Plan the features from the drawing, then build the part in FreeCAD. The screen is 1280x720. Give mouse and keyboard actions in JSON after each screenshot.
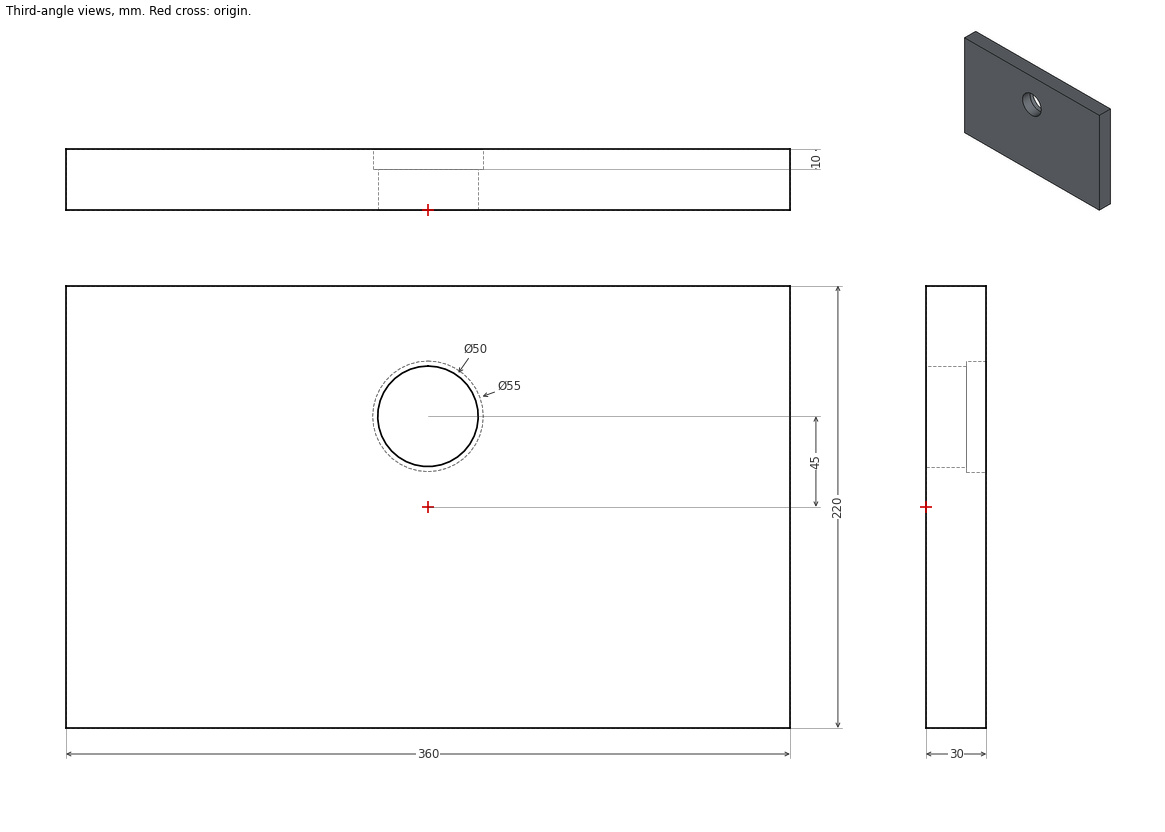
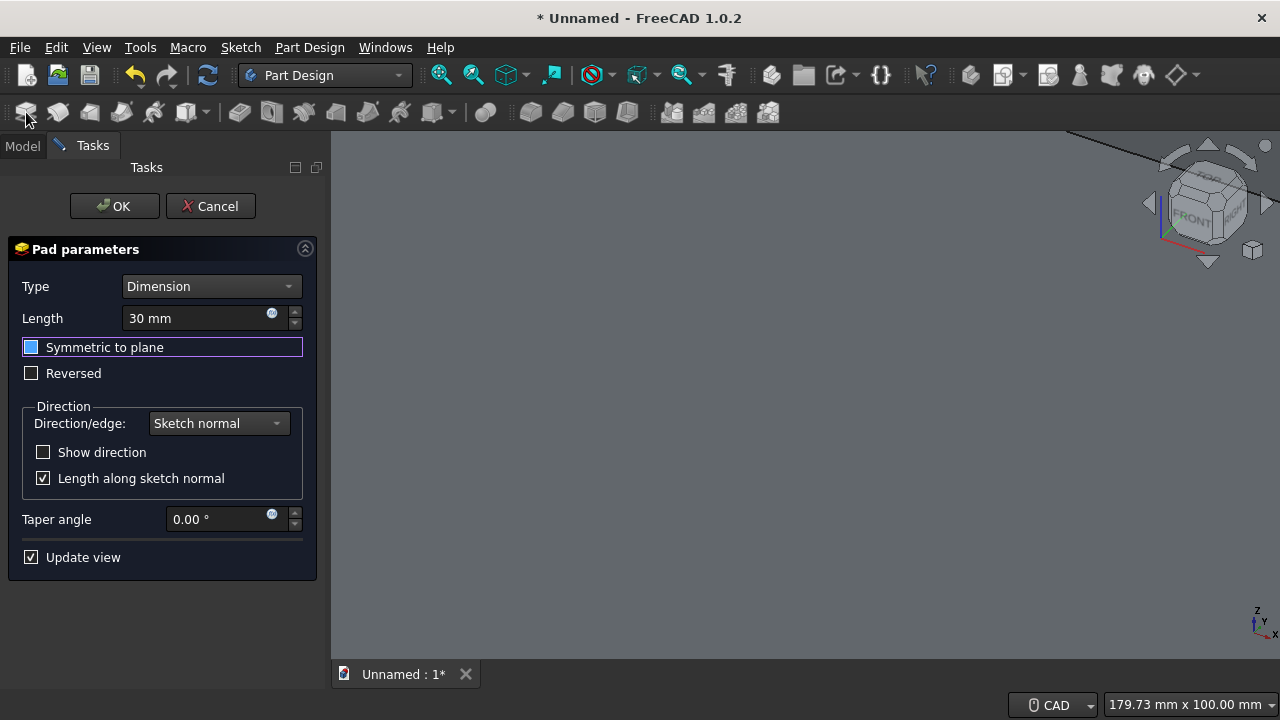
{"action": "left_click", "coordinate": [30, 373]}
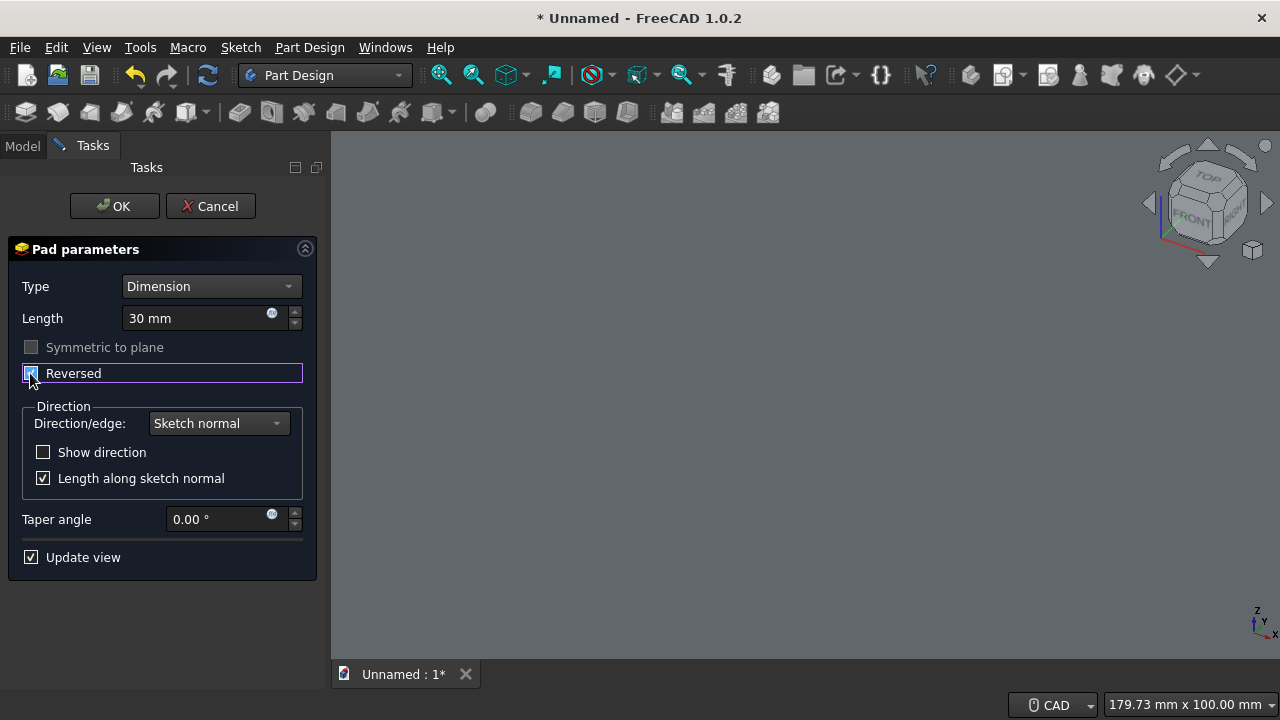
{"action": "left_click", "coordinate": [115, 206]}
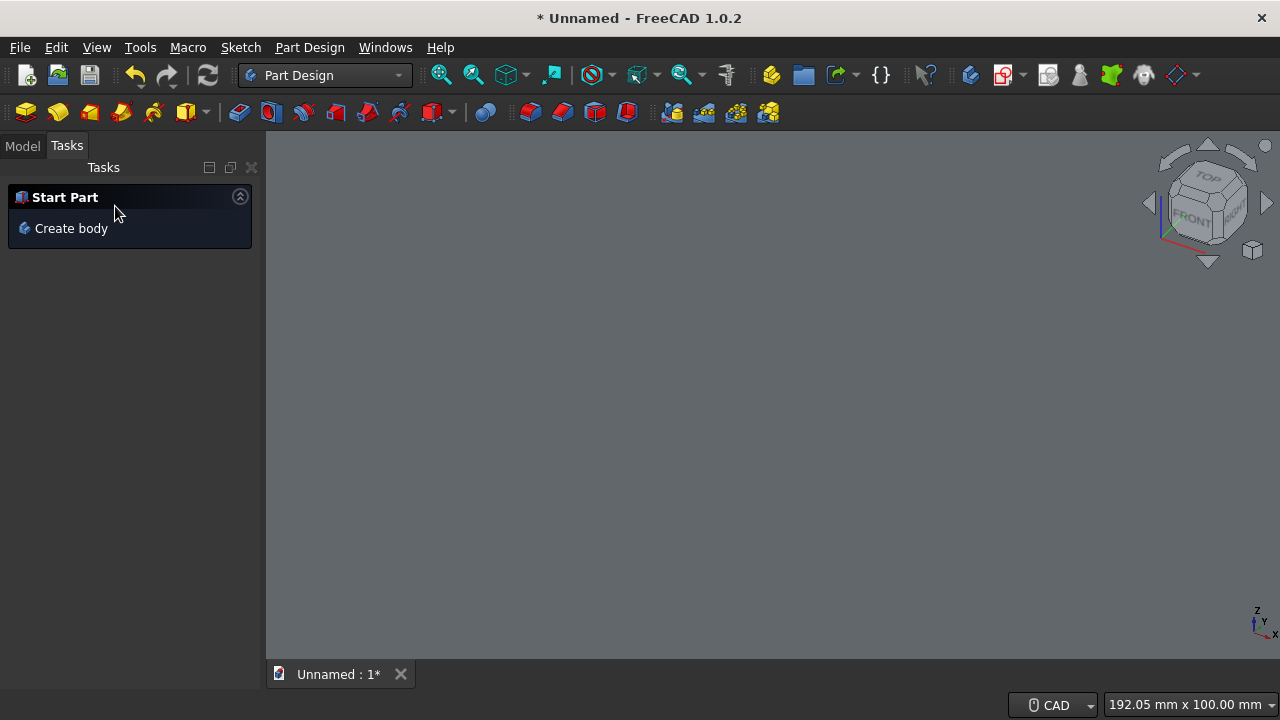
{"action": "key", "text": "v f"}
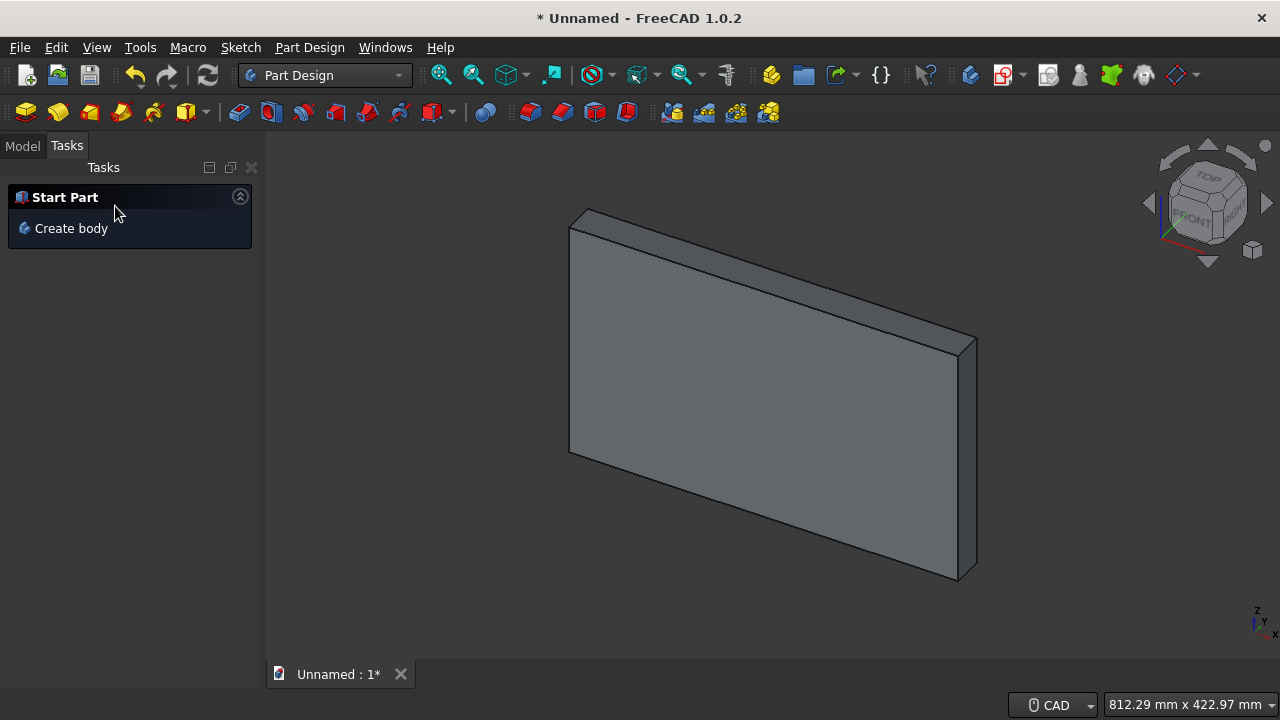
{"action": "key", "text": "4"}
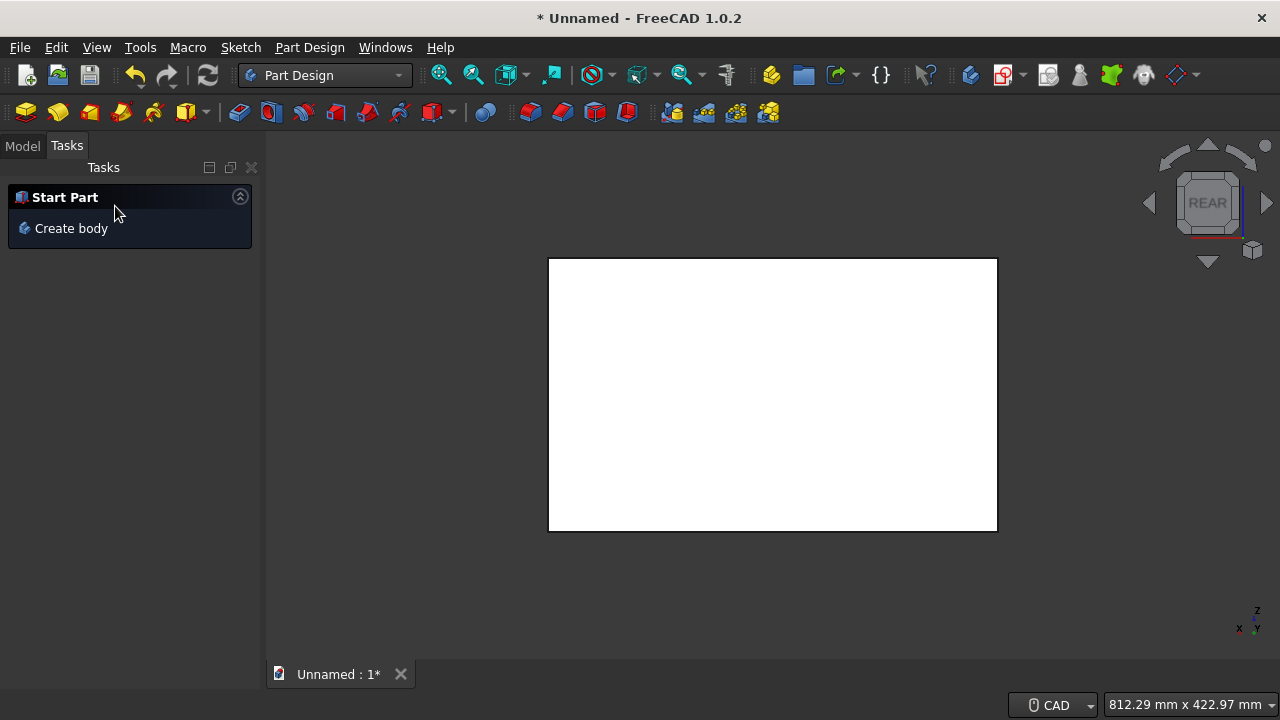
{"action": "left_click", "coordinate": [709, 394]}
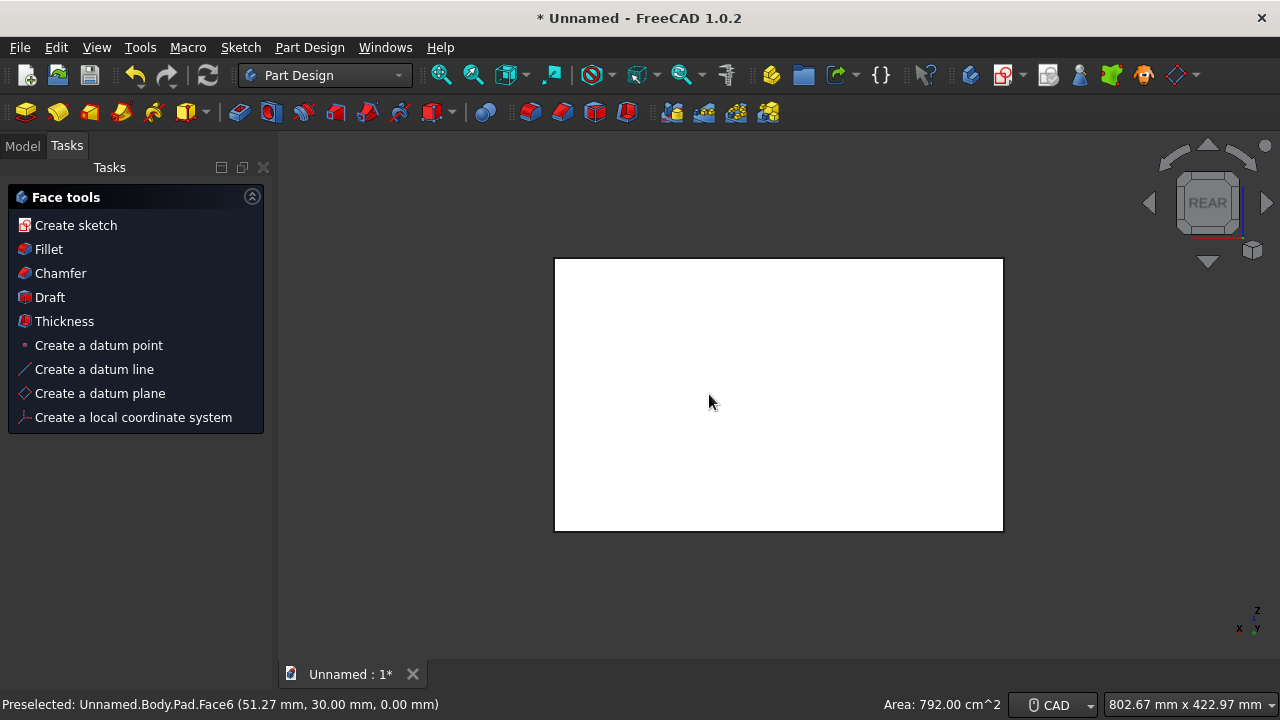
{"action": "left_click", "coordinate": [1004, 76]}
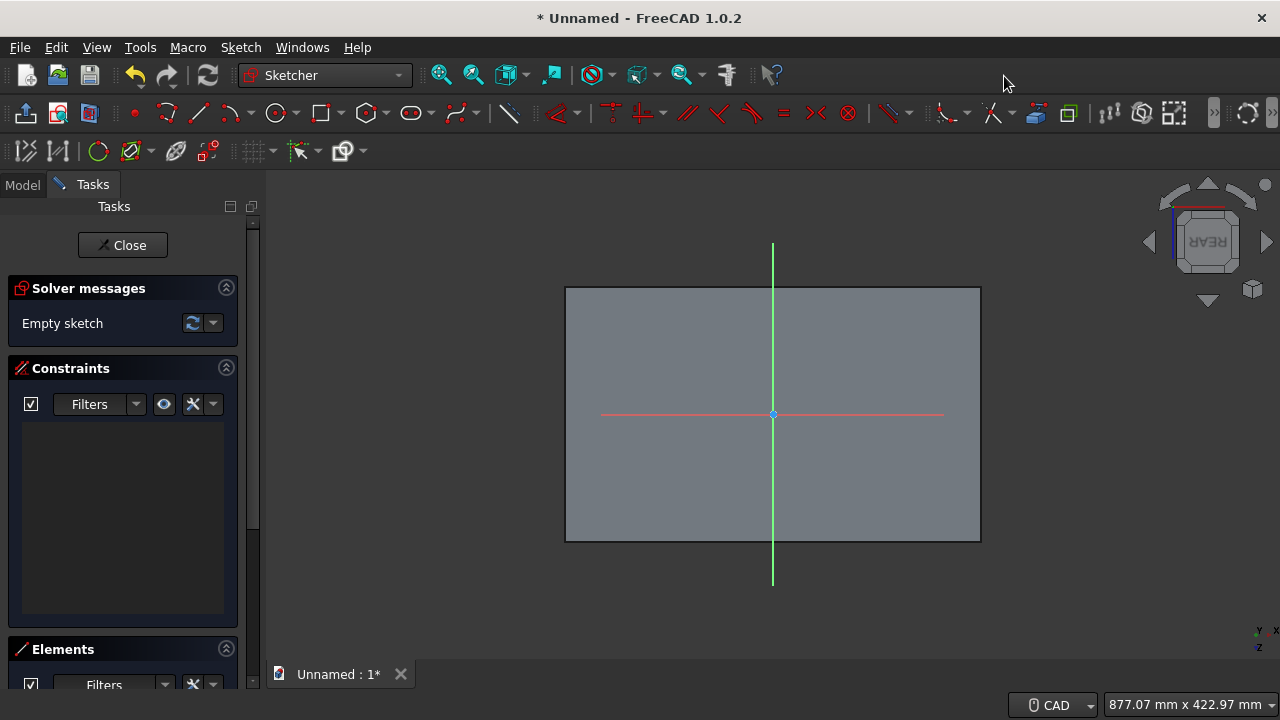
{"action": "scroll", "coordinate": [803, 474], "scroll_direction": "up", "scroll_amount": 6}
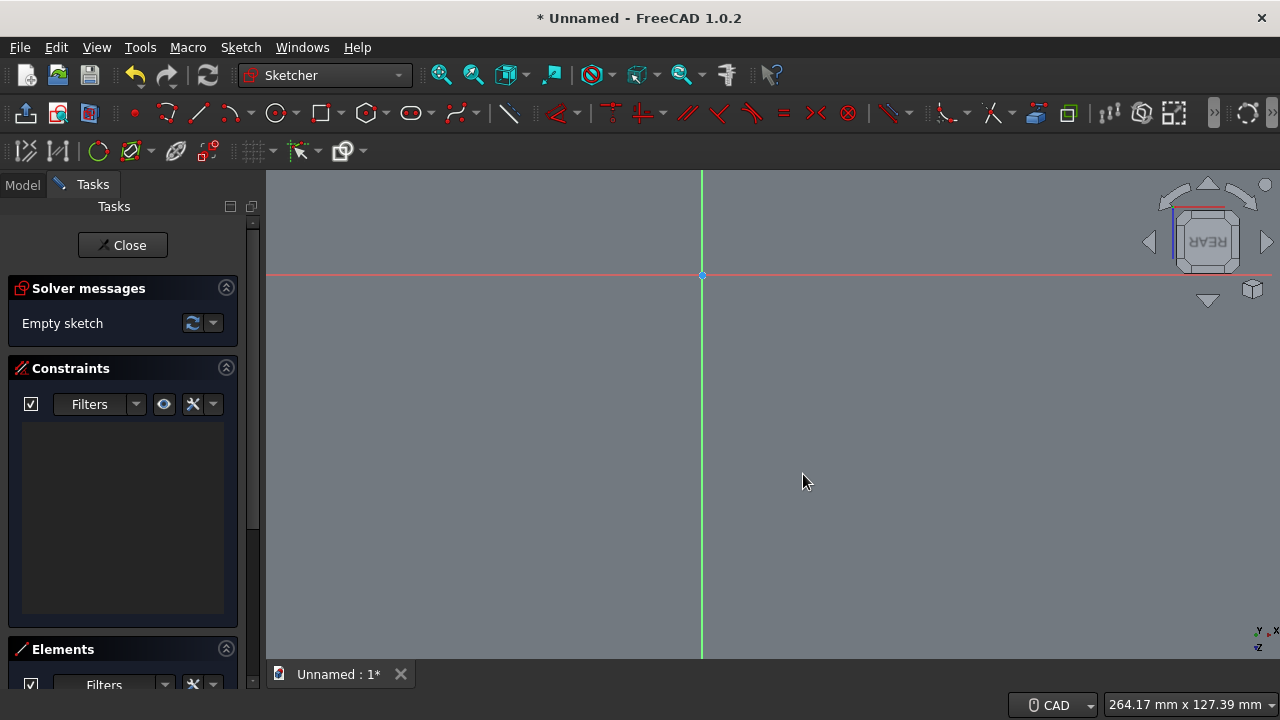
{"action": "key", "text": "g c"}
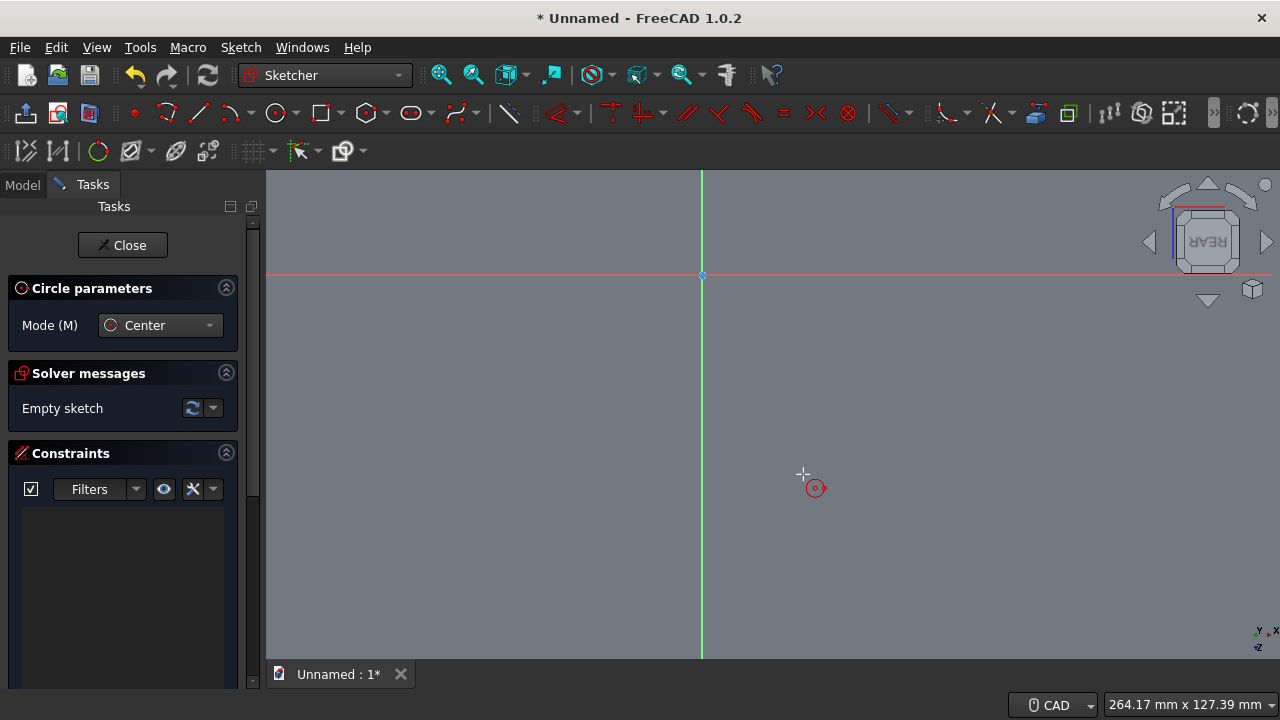
{"action": "left_click", "coordinate": [702, 448]}
{"action": "mouse_move", "coordinate": [777, 373]}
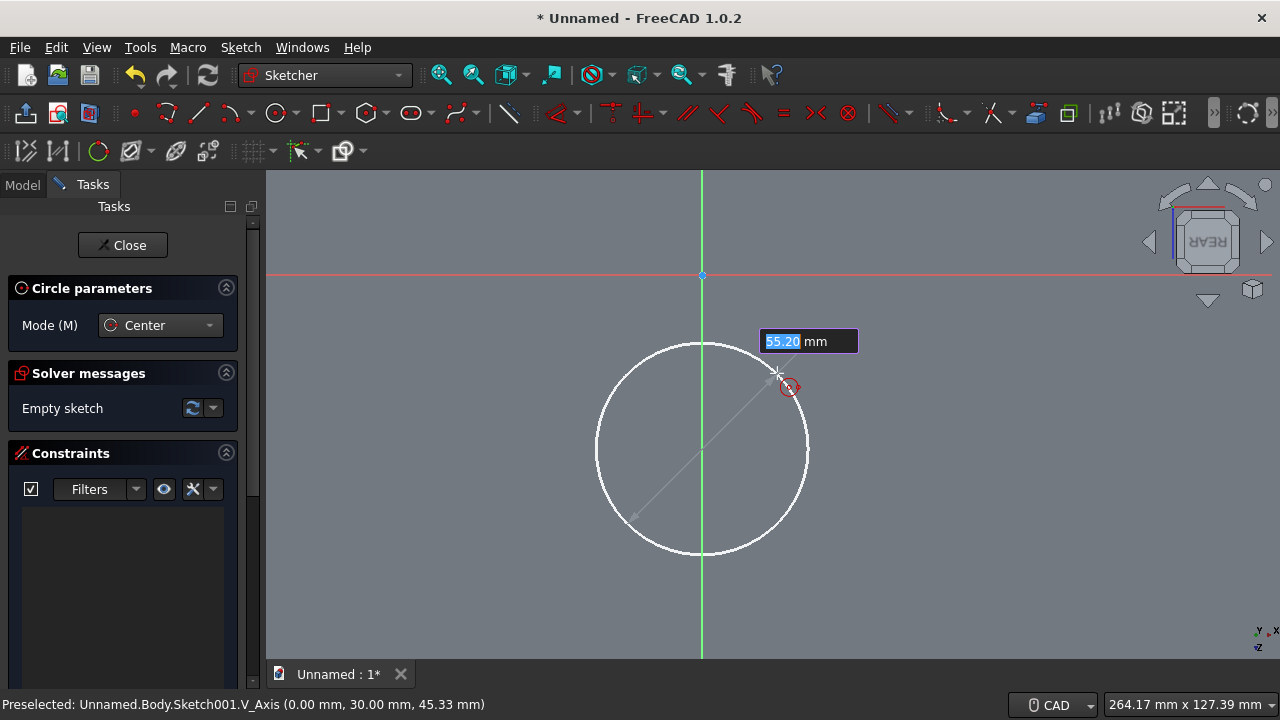
{"action": "type", "text": "55"}
{"action": "key", "text": "Return"}
{"action": "key", "text": "Escape"}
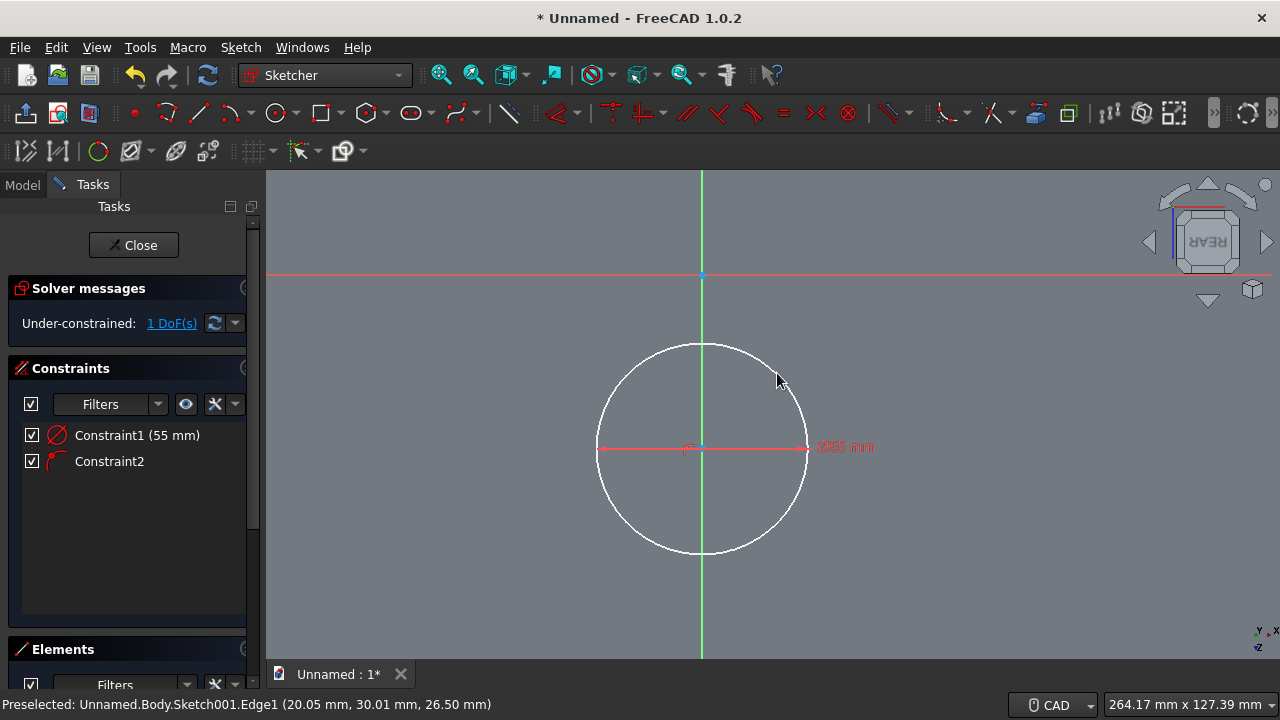
{"action": "left_click", "coordinate": [556, 114]}